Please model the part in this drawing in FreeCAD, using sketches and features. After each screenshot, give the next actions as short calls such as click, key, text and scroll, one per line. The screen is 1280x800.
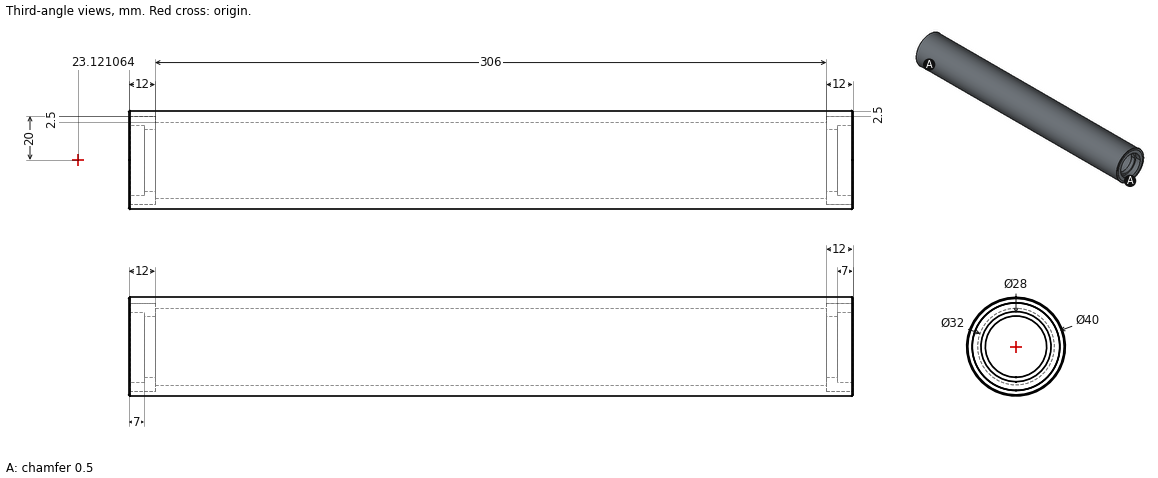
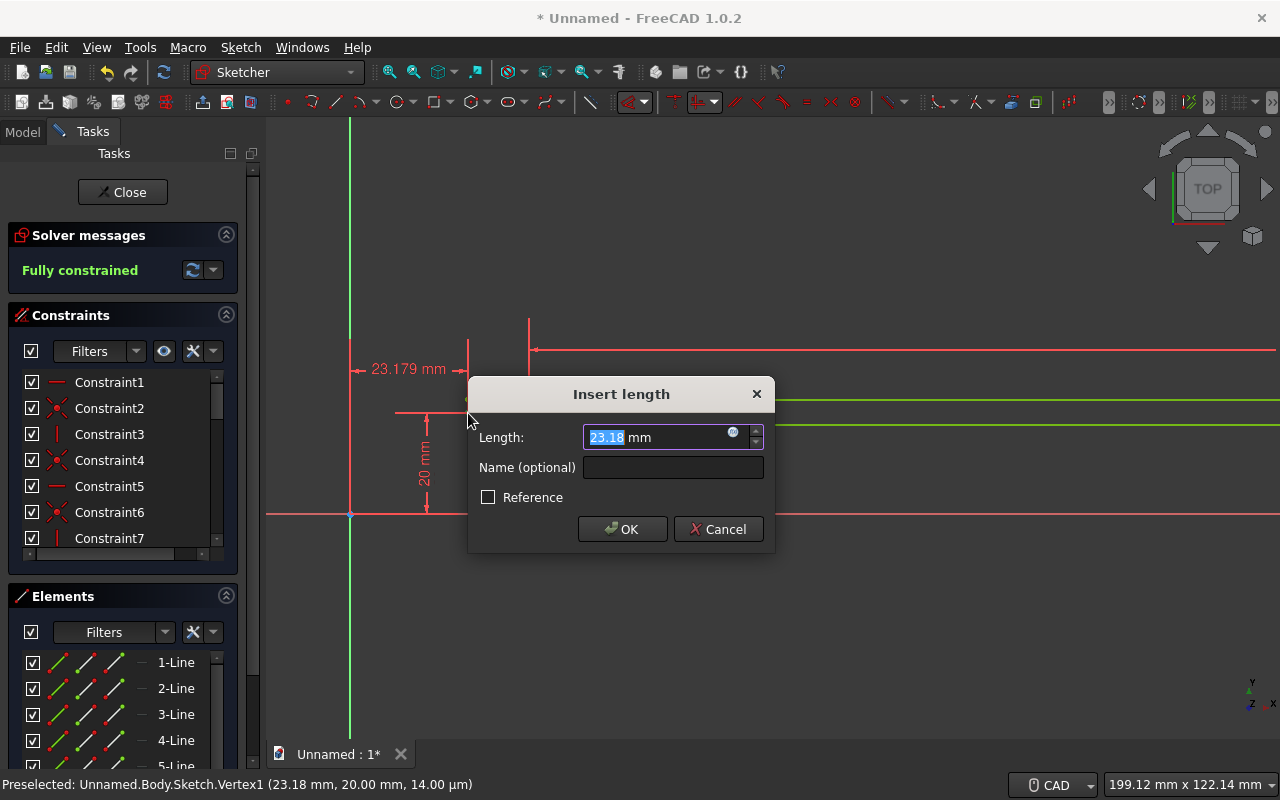
text(23.121064)
key(Return)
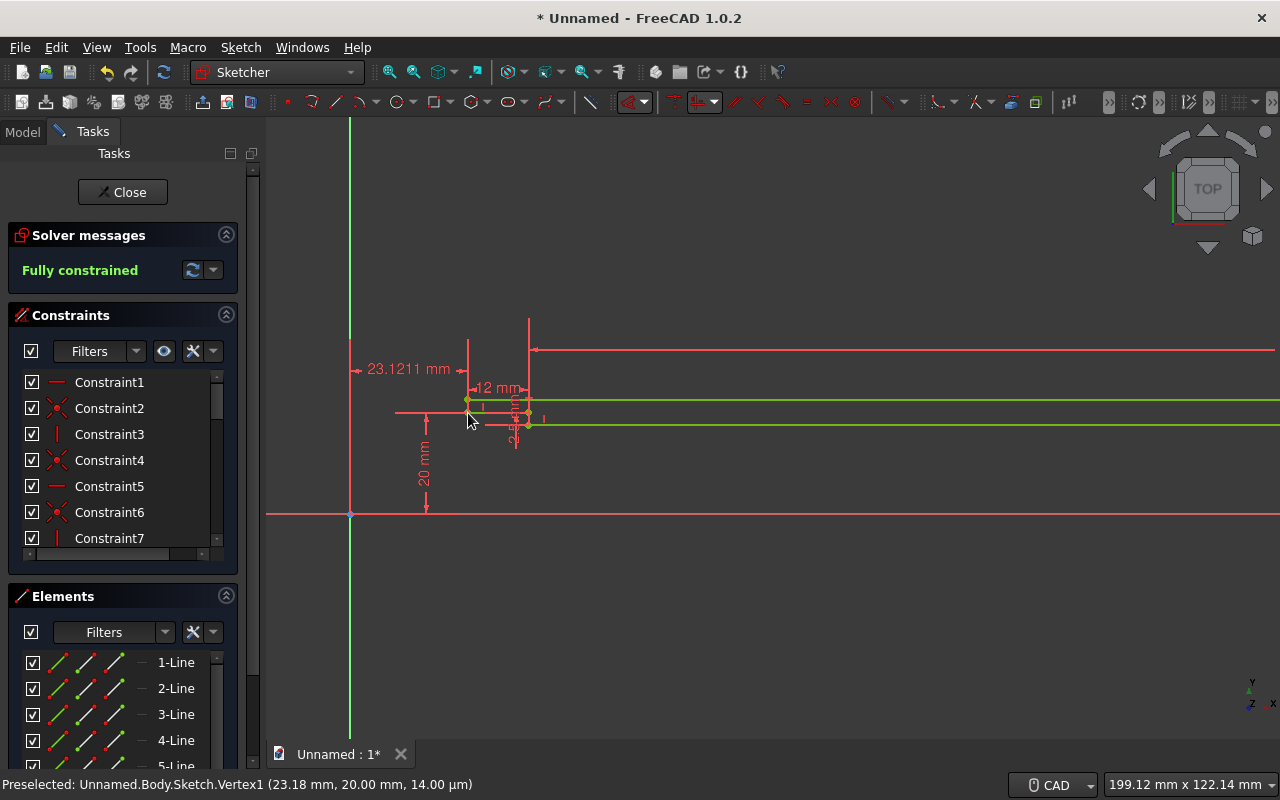
click(123, 192)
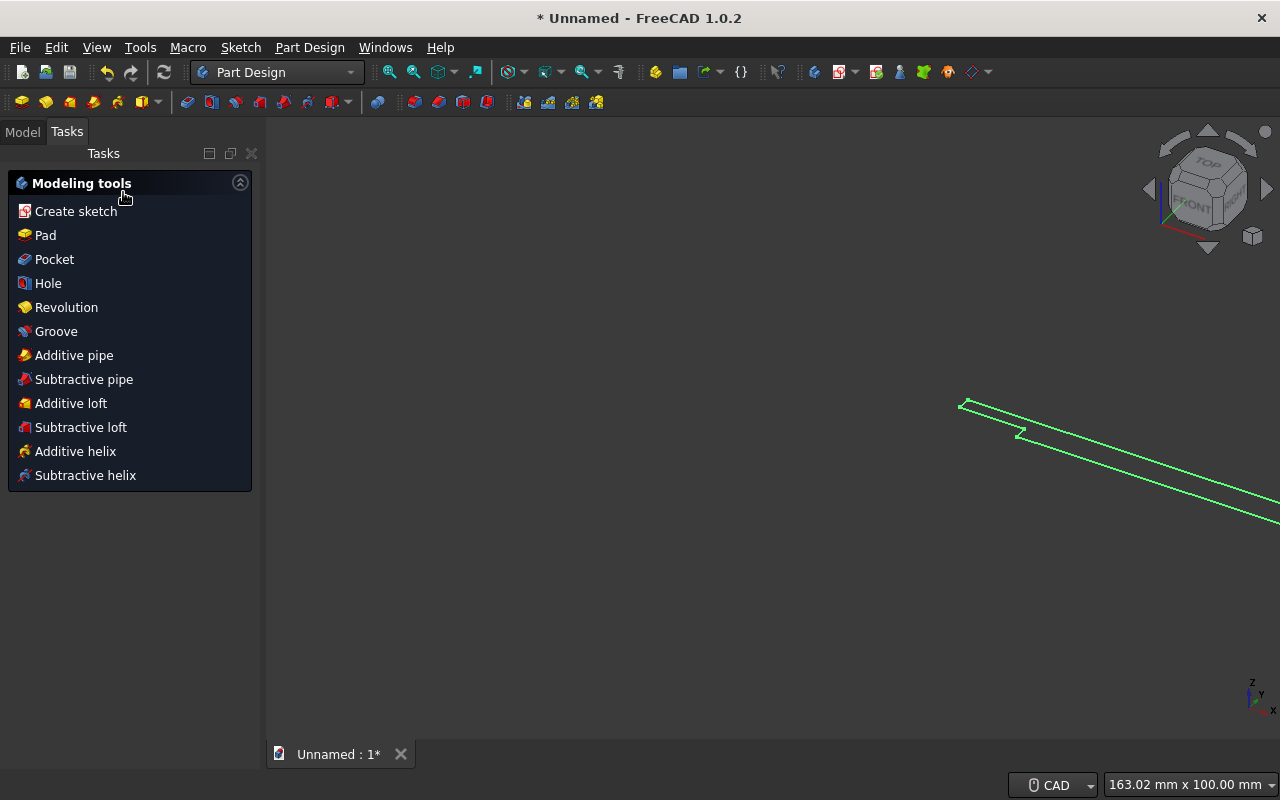
click(46, 102)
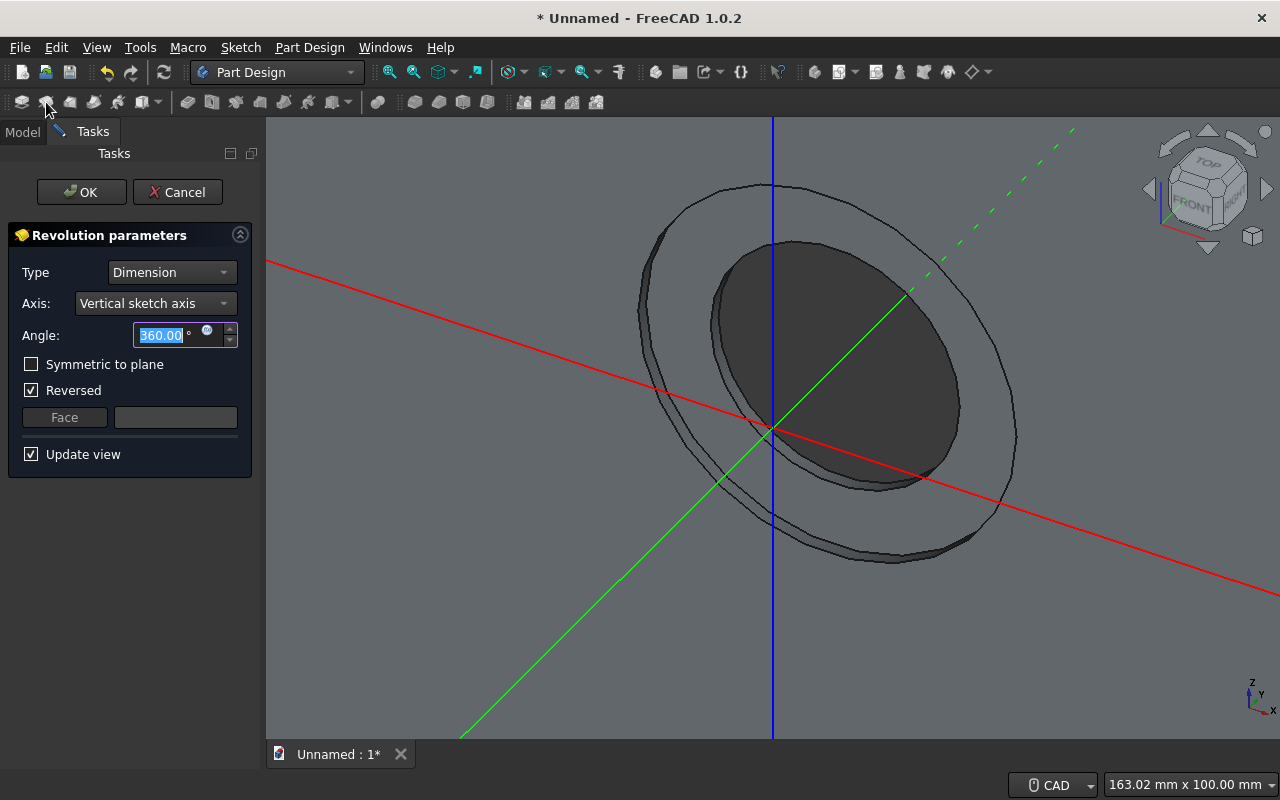
click(156, 304)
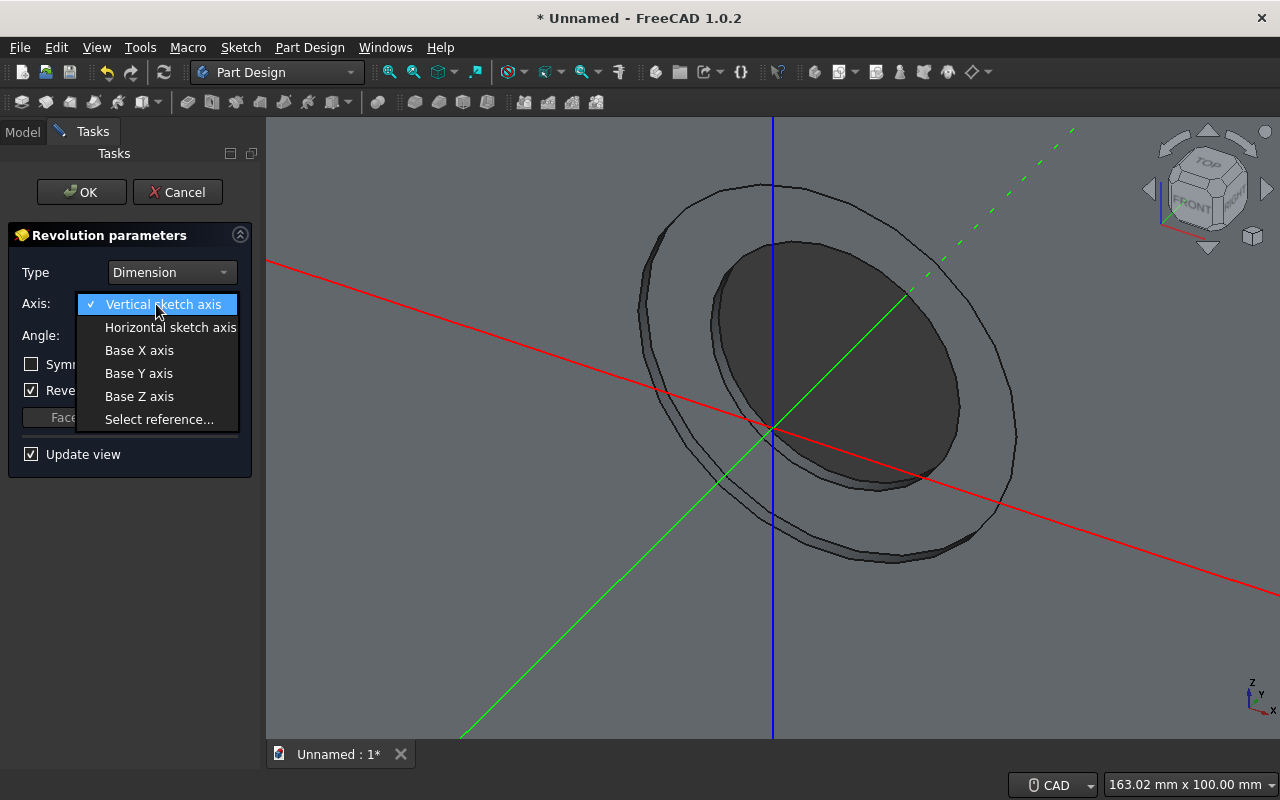
click(156, 328)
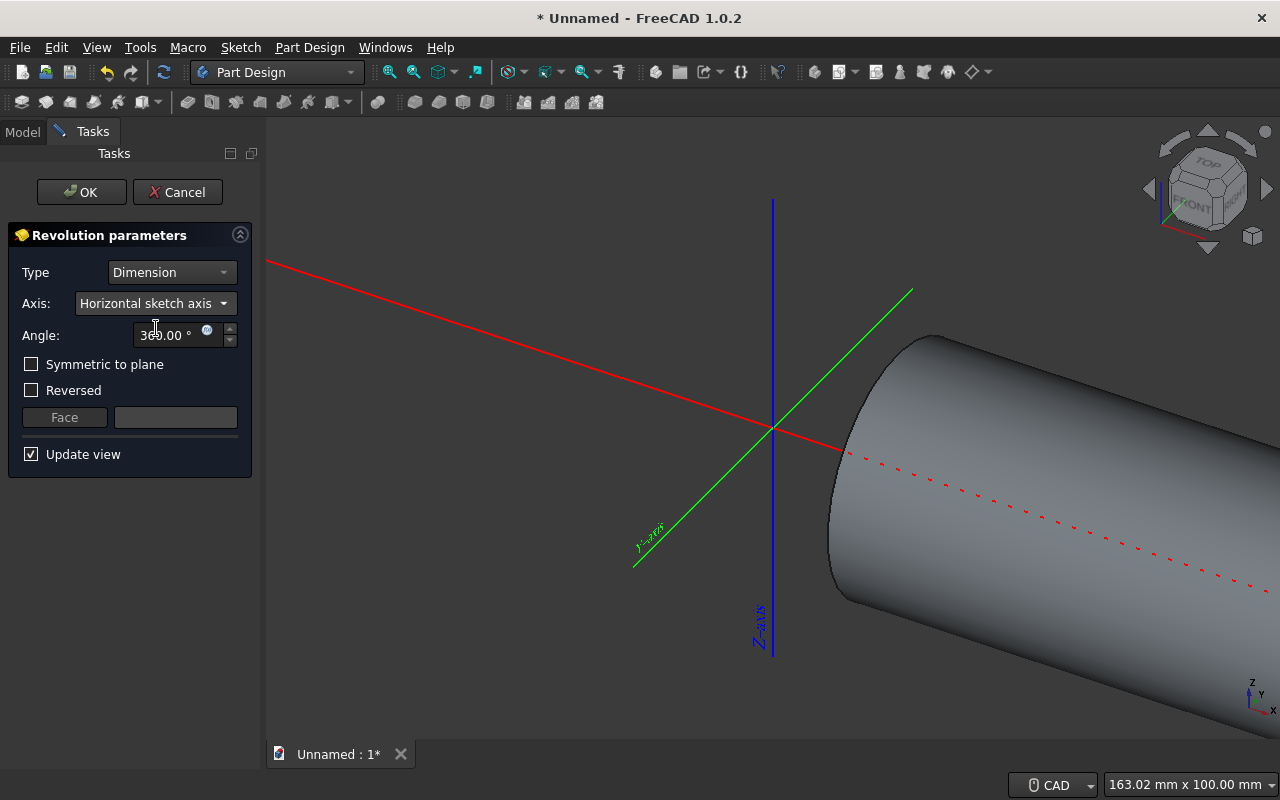
click(82, 192)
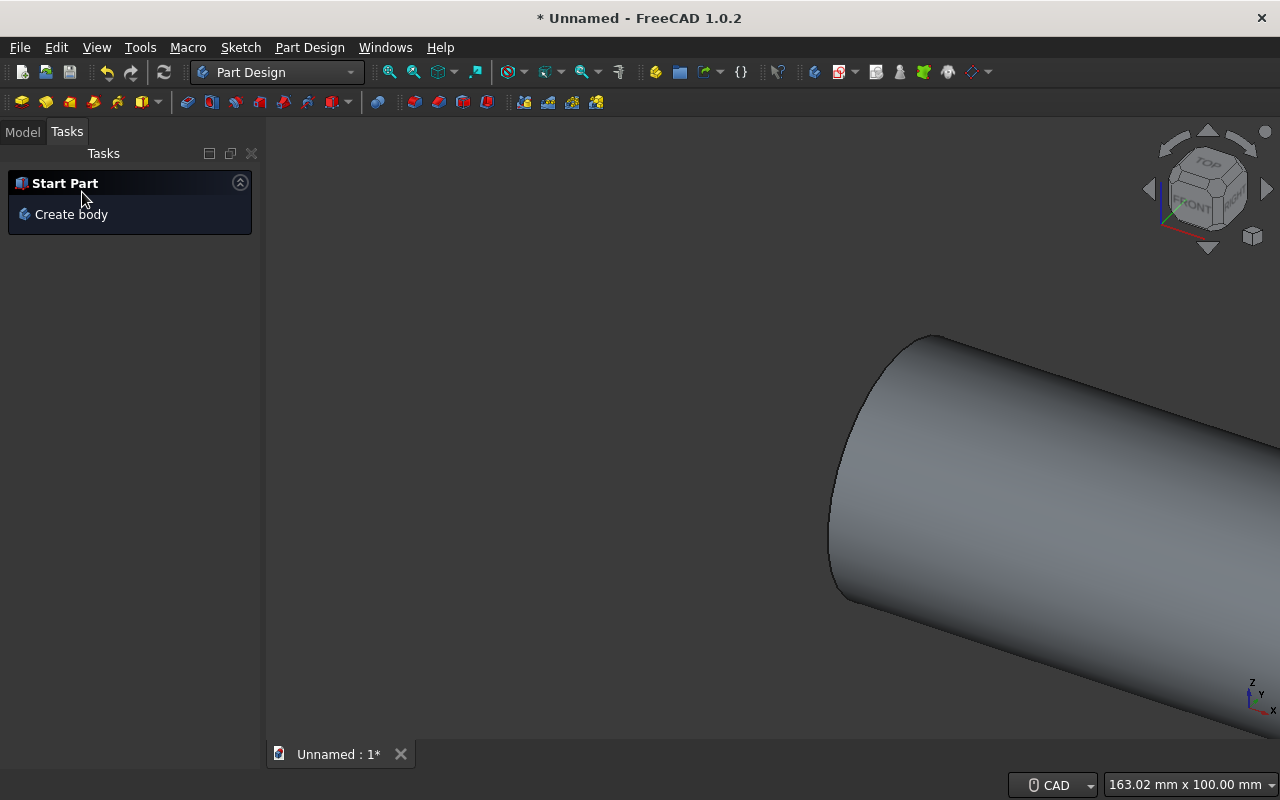
click(390, 72)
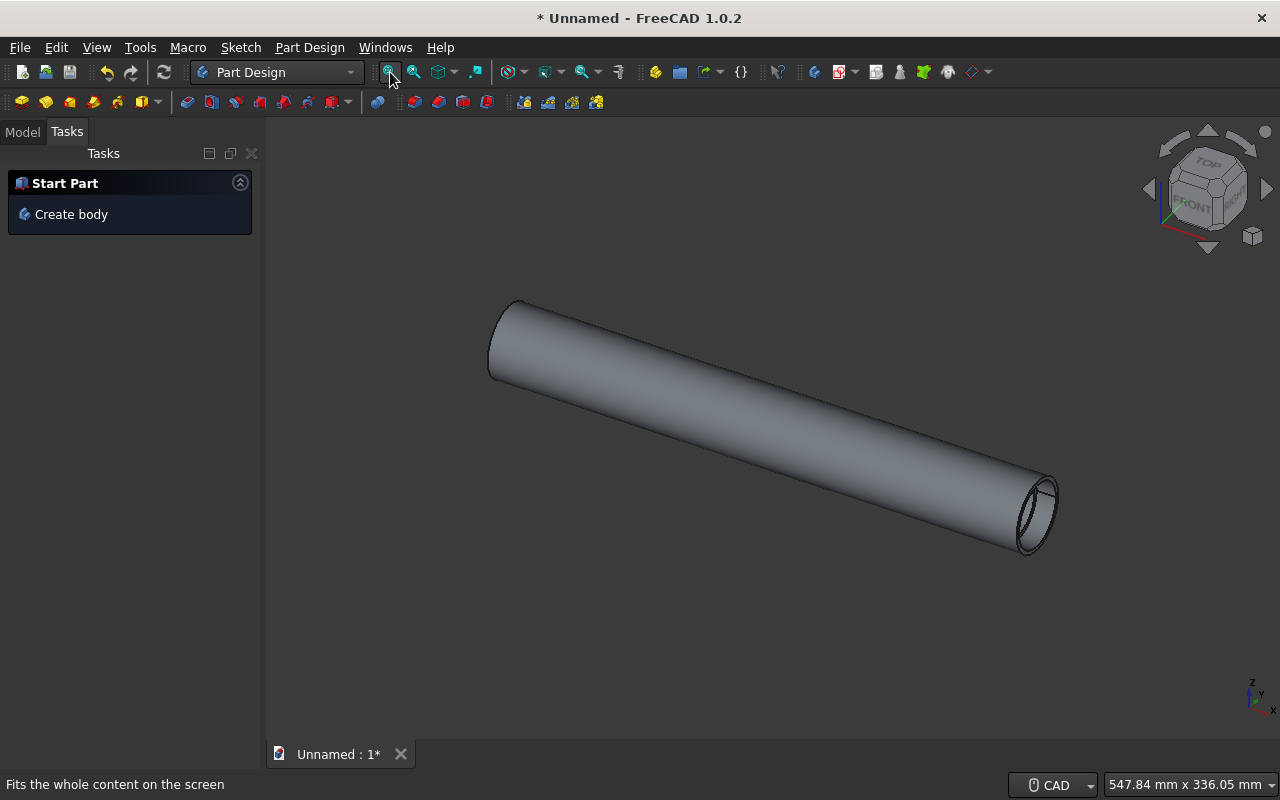
click(1017, 535)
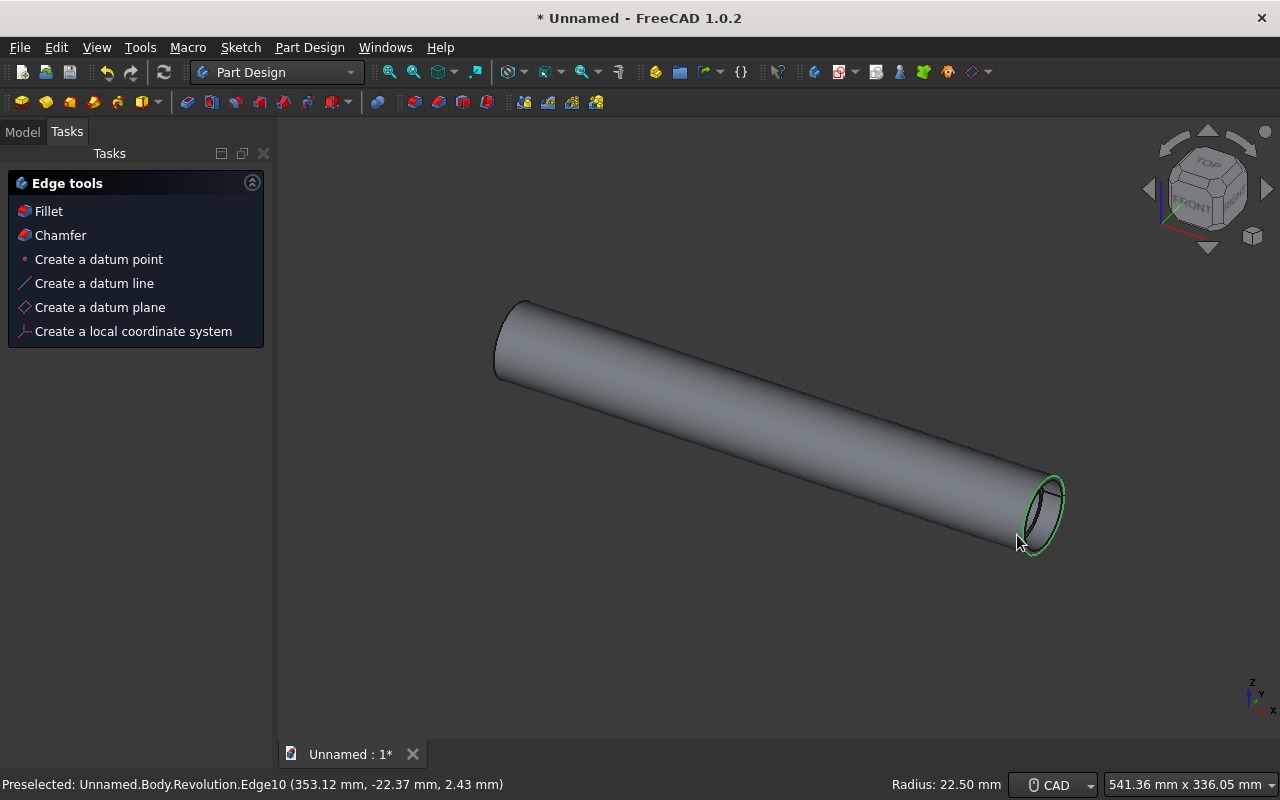
click(508, 313, ctrl)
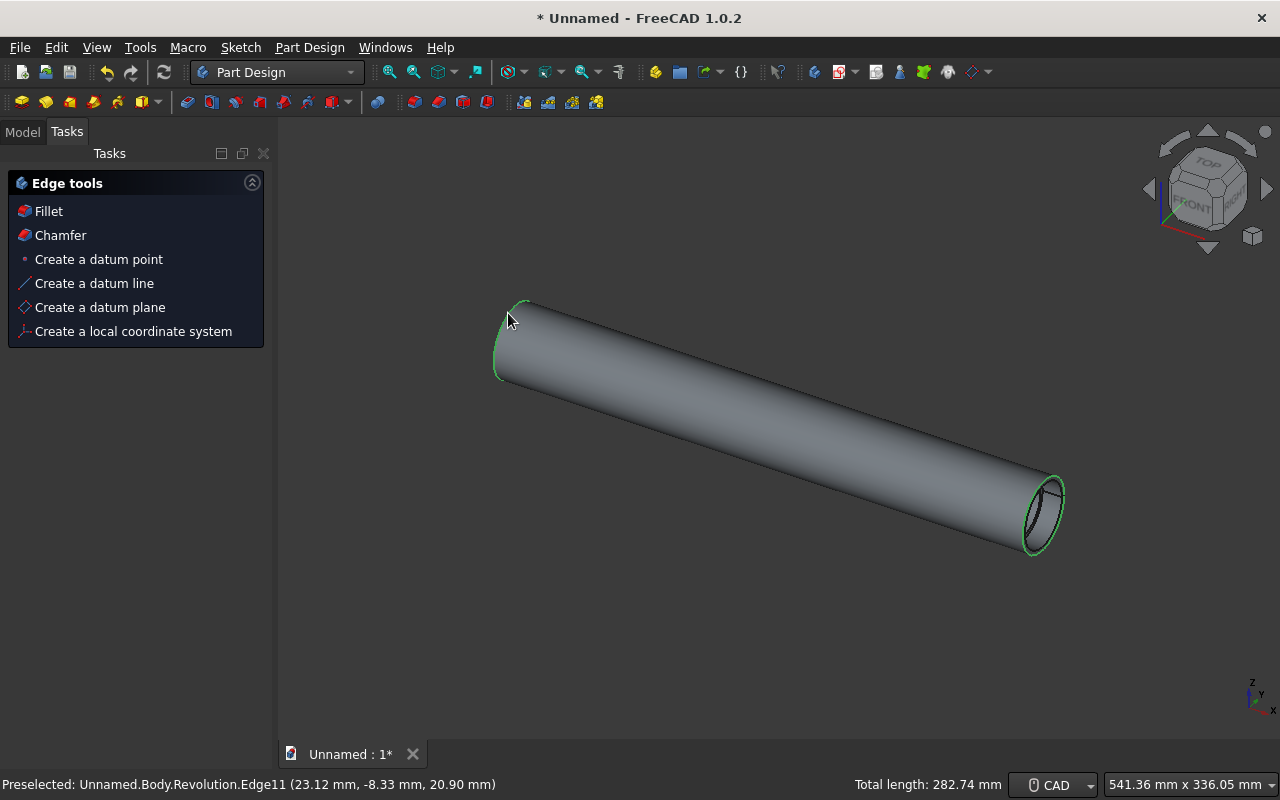
click(440, 102)